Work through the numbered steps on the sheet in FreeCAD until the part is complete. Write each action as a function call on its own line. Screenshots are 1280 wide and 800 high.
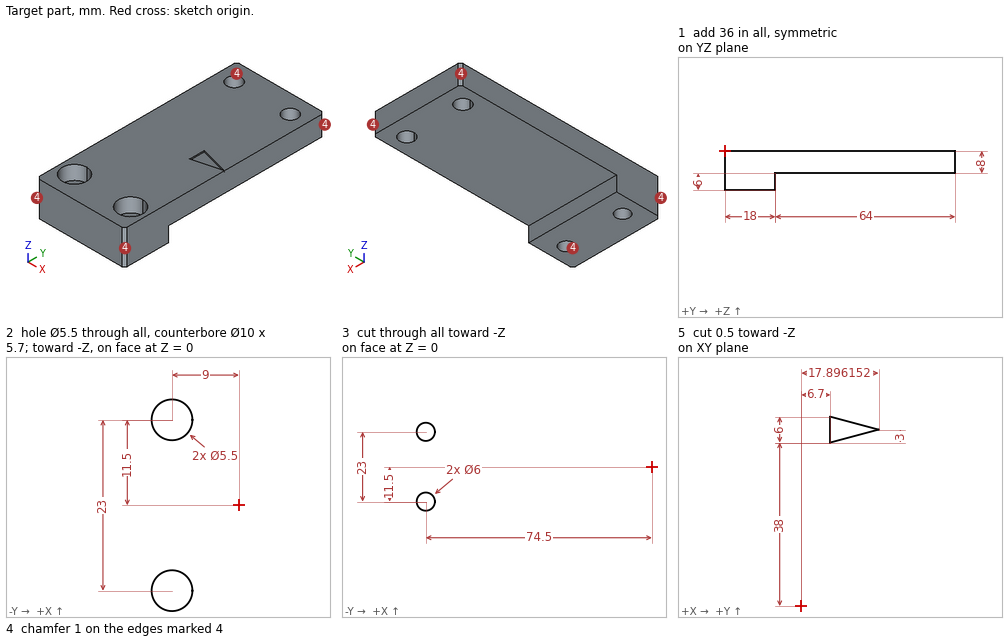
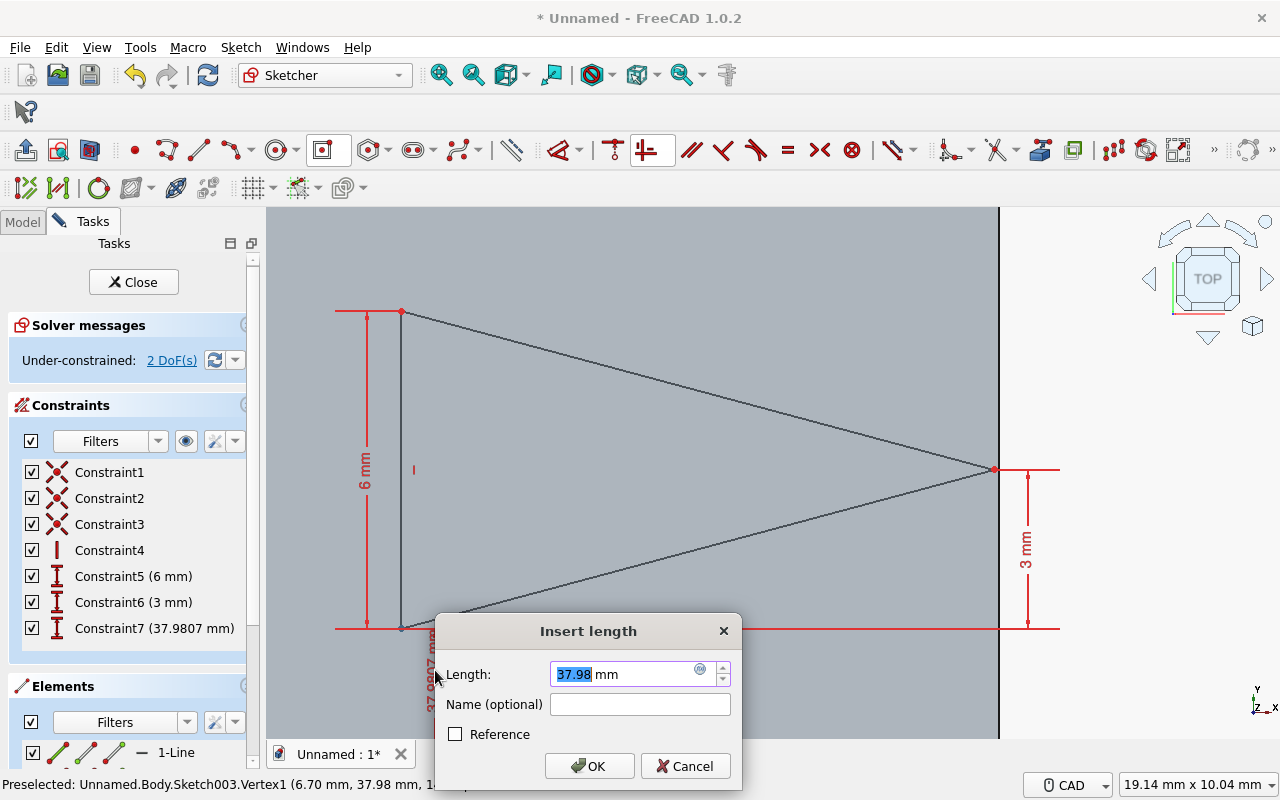
text(38)
key(Return)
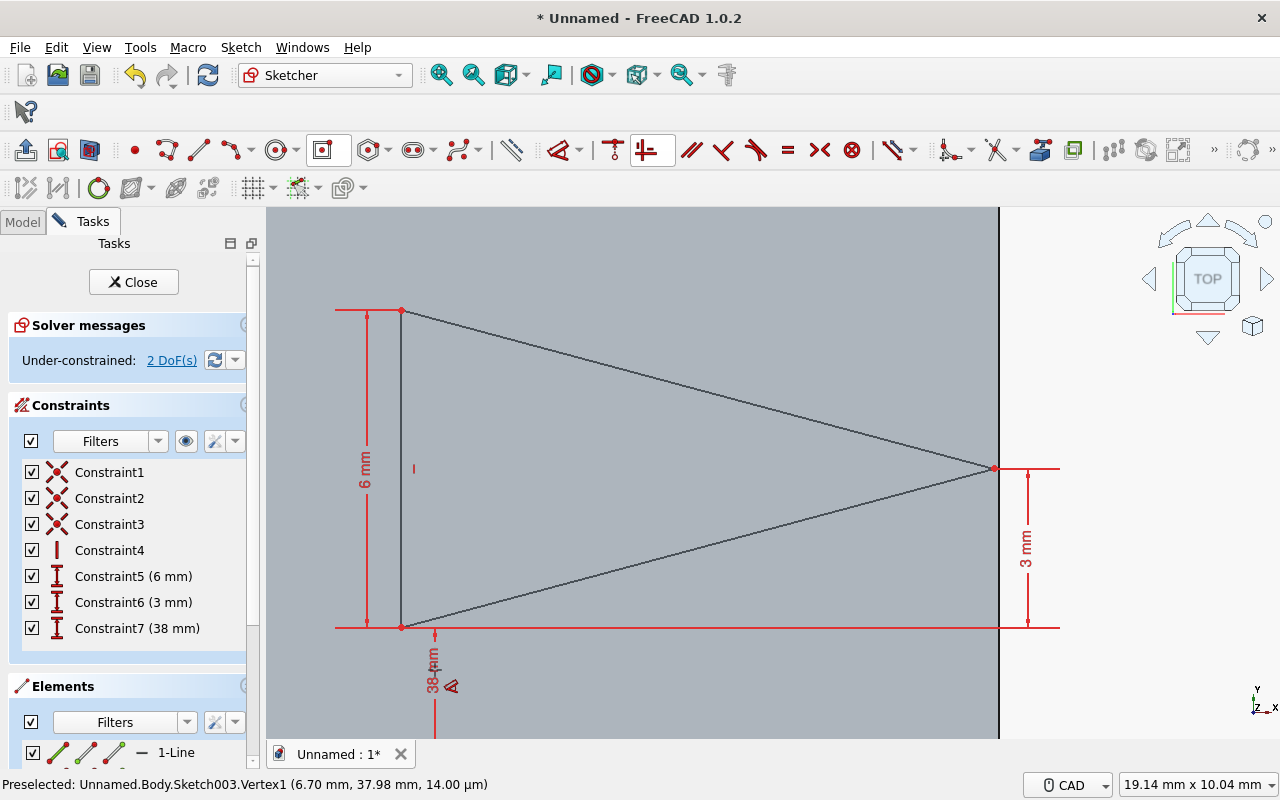
click(401, 628)
click(347, 594)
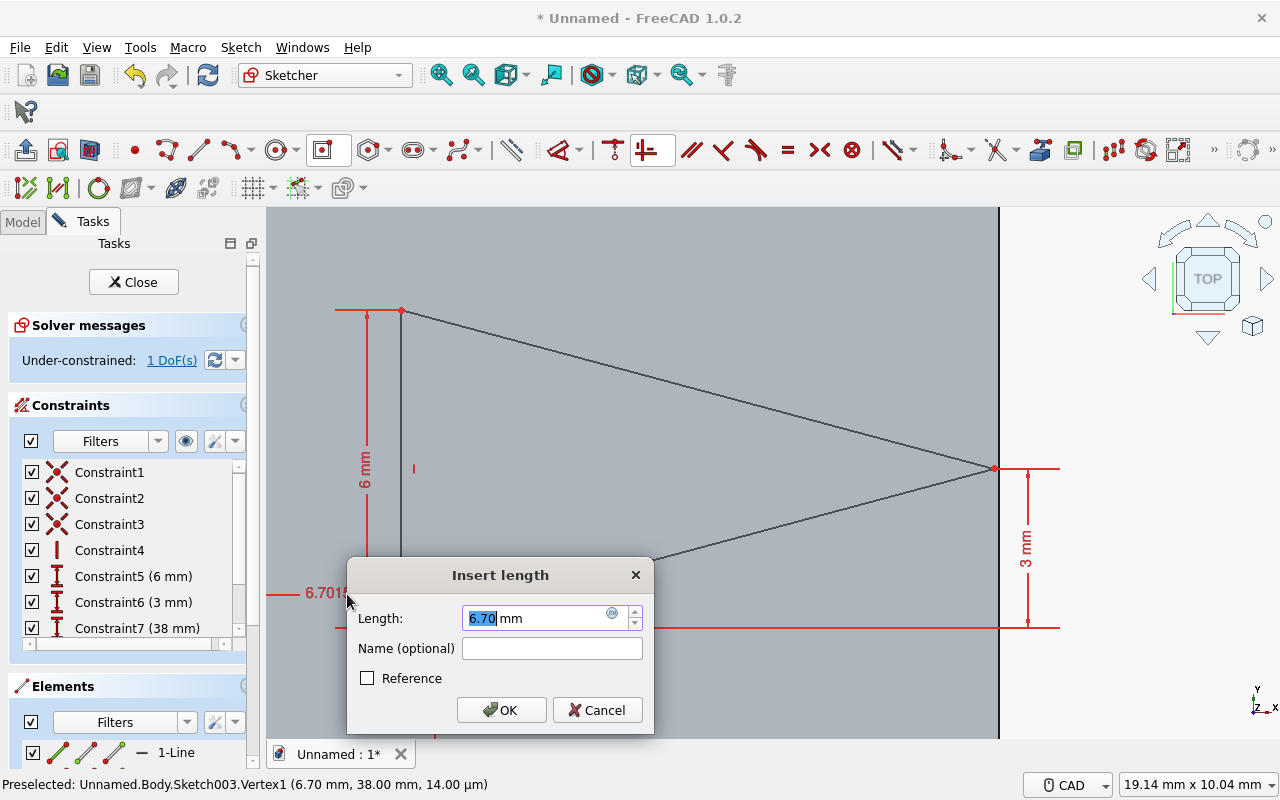
text(6.7)
key(Return)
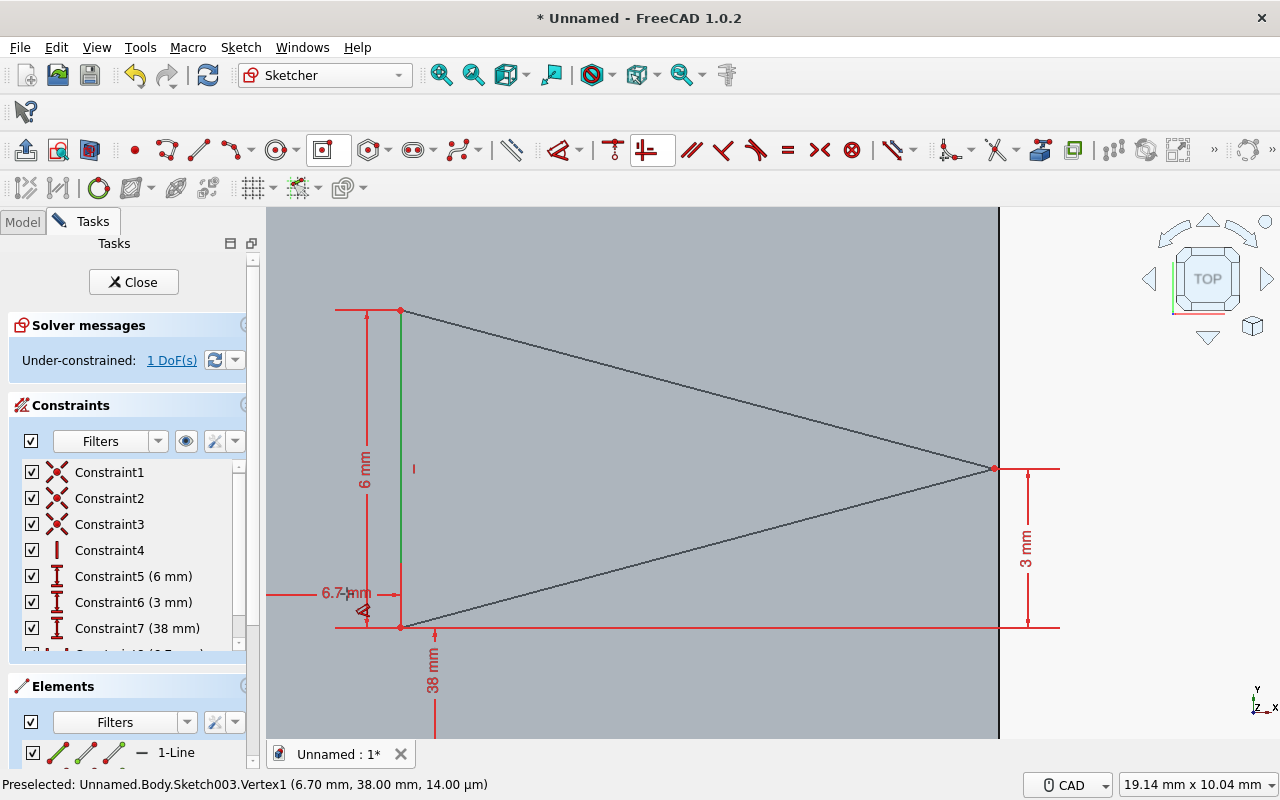
click(994, 469)
click(644, 435)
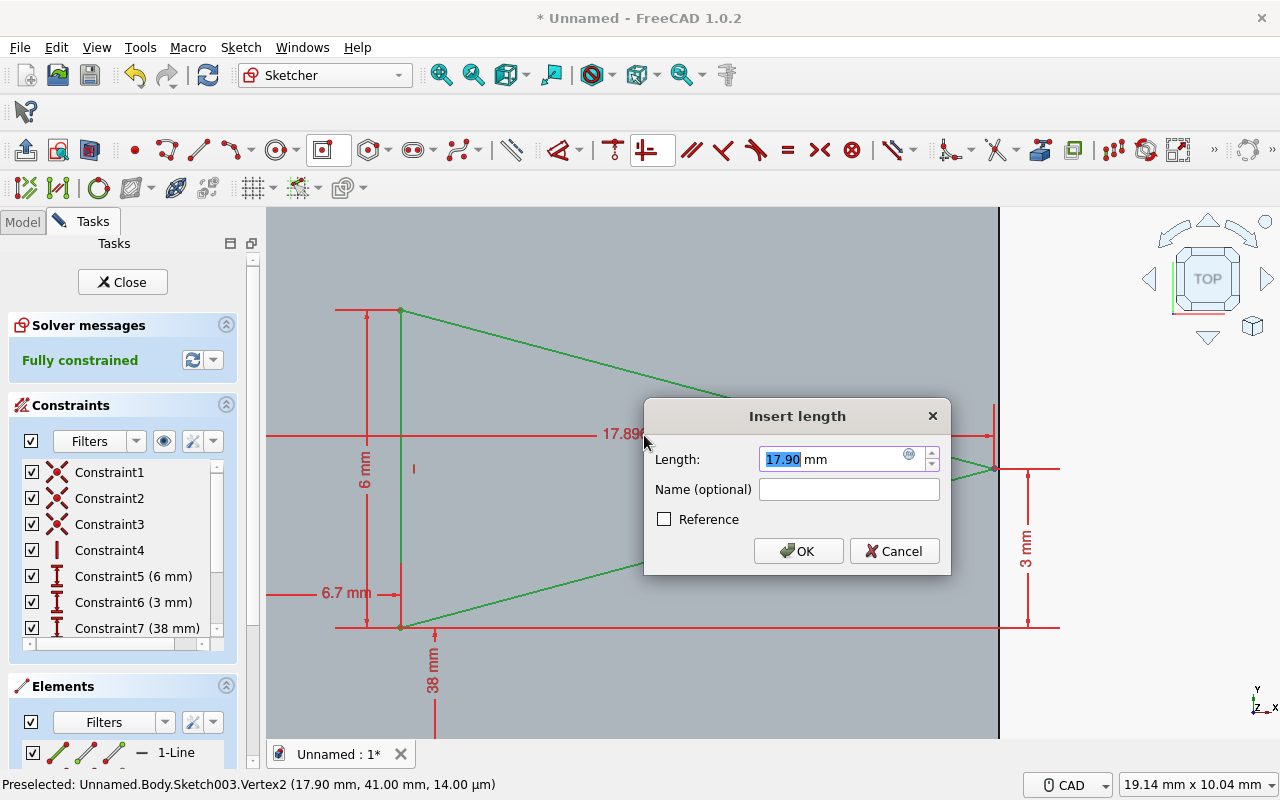
text(17.896152)
key(Return)
key(Escape)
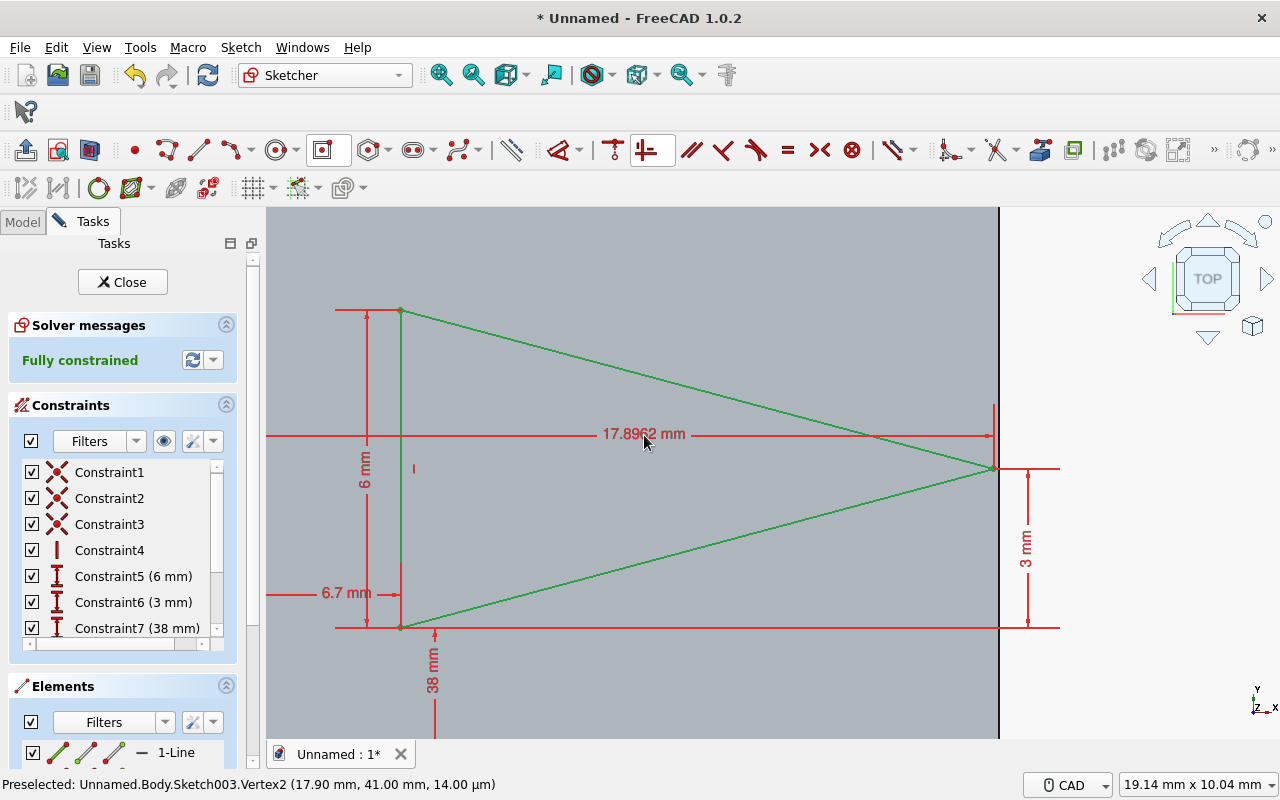
click(123, 282)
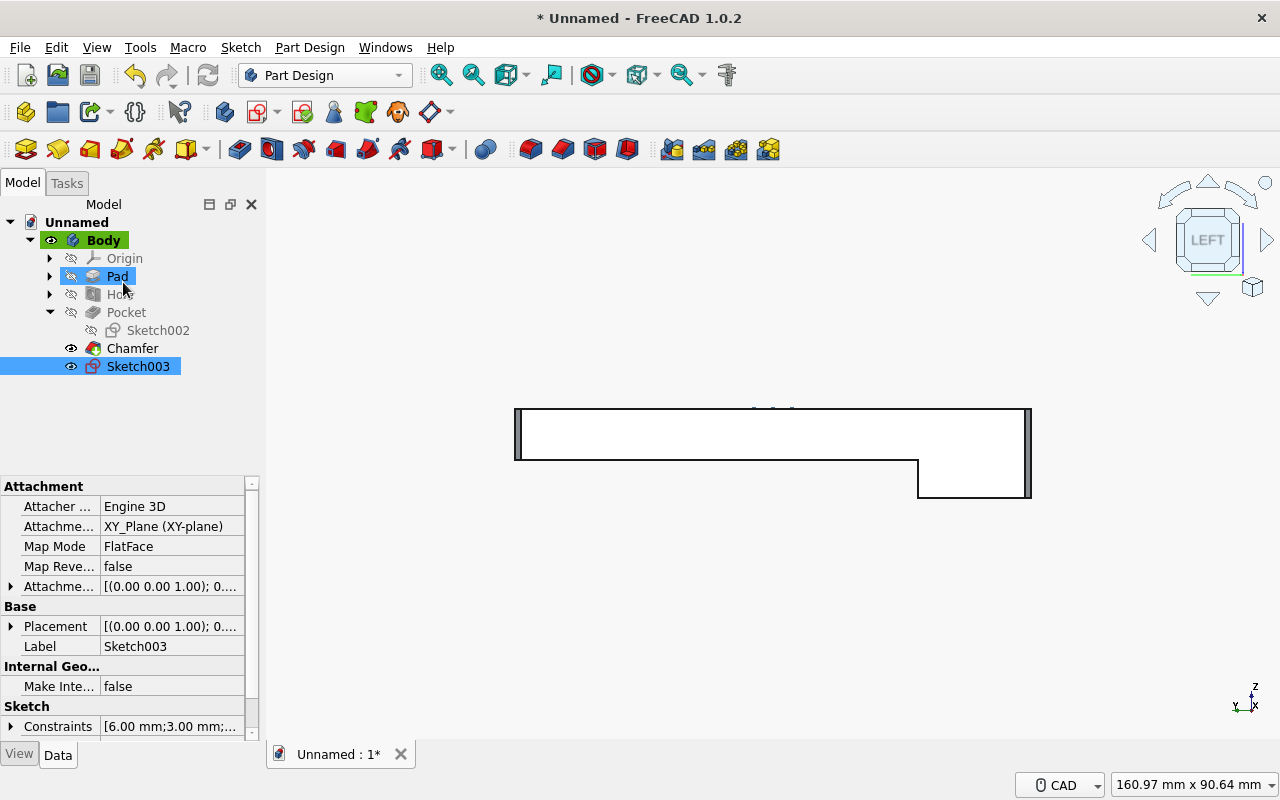
click(240, 150)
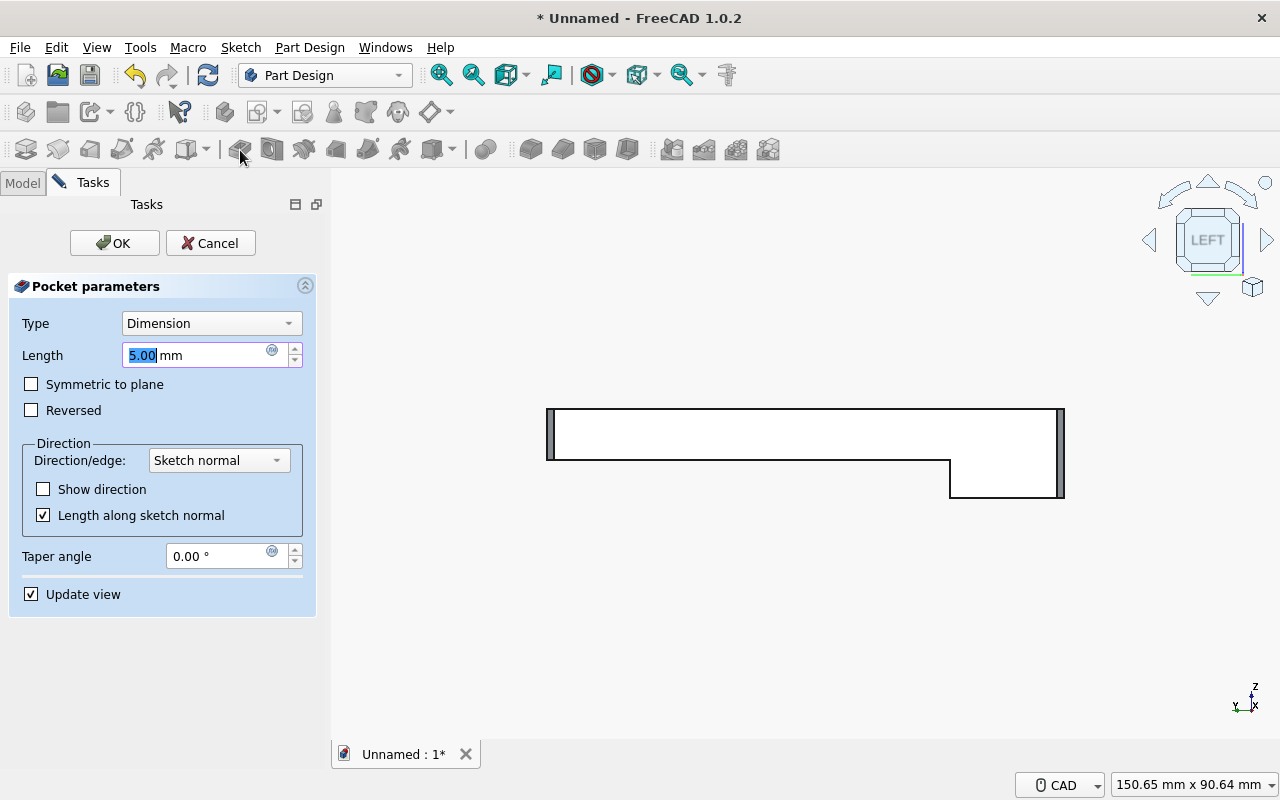
text(0.5)
key(Tab)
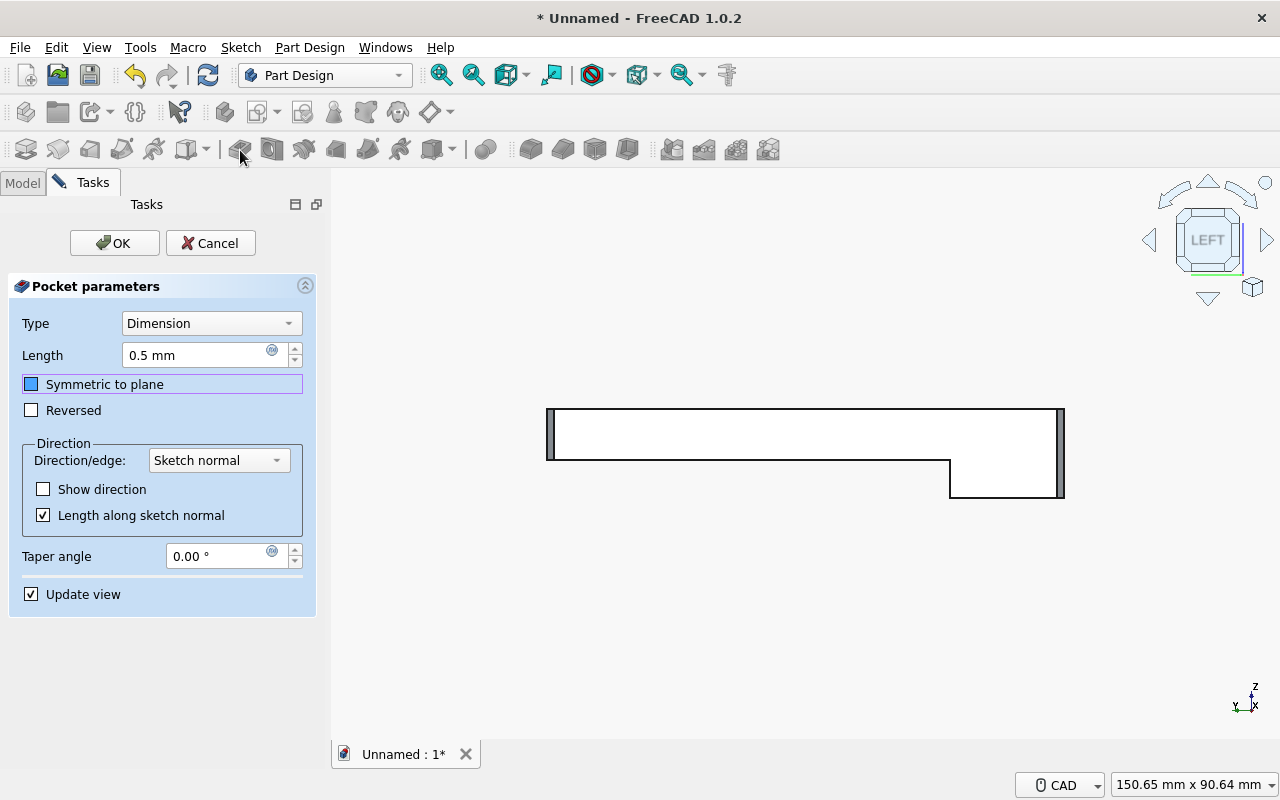
click(115, 243)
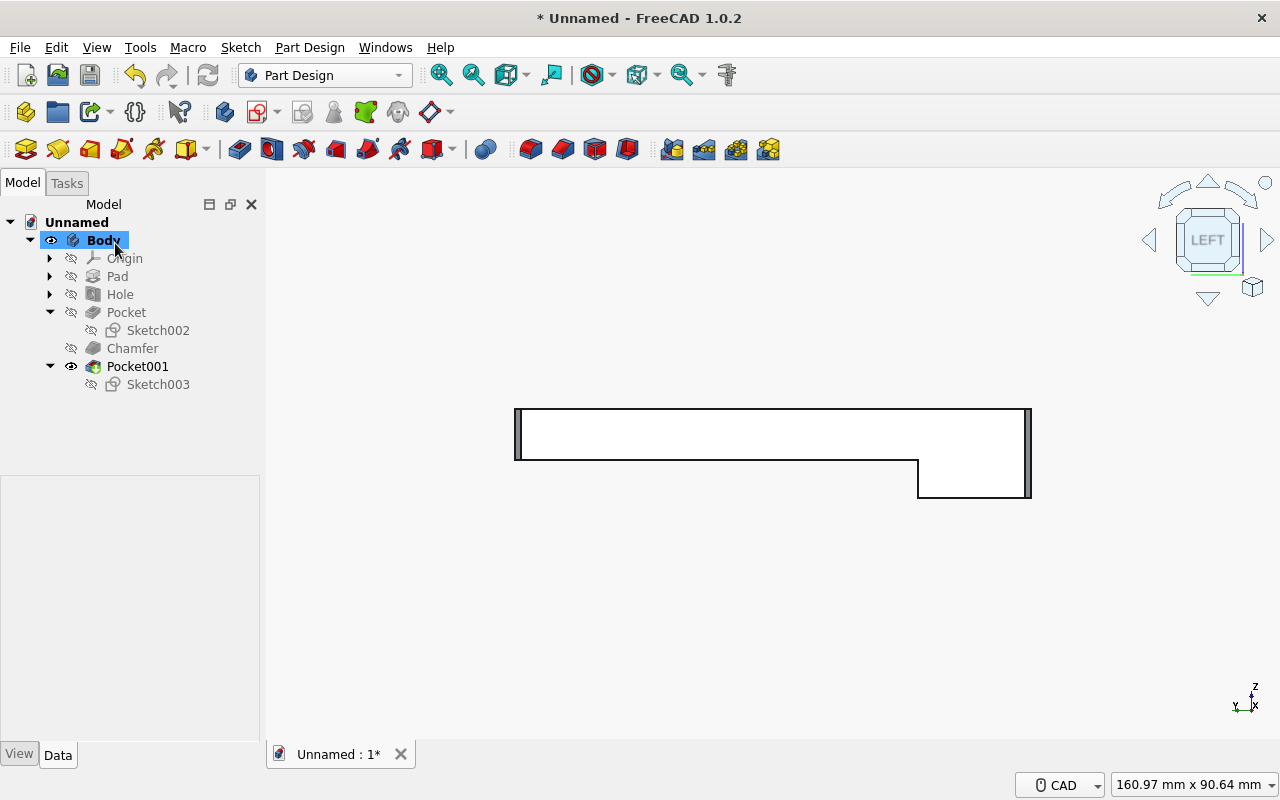
key(0)